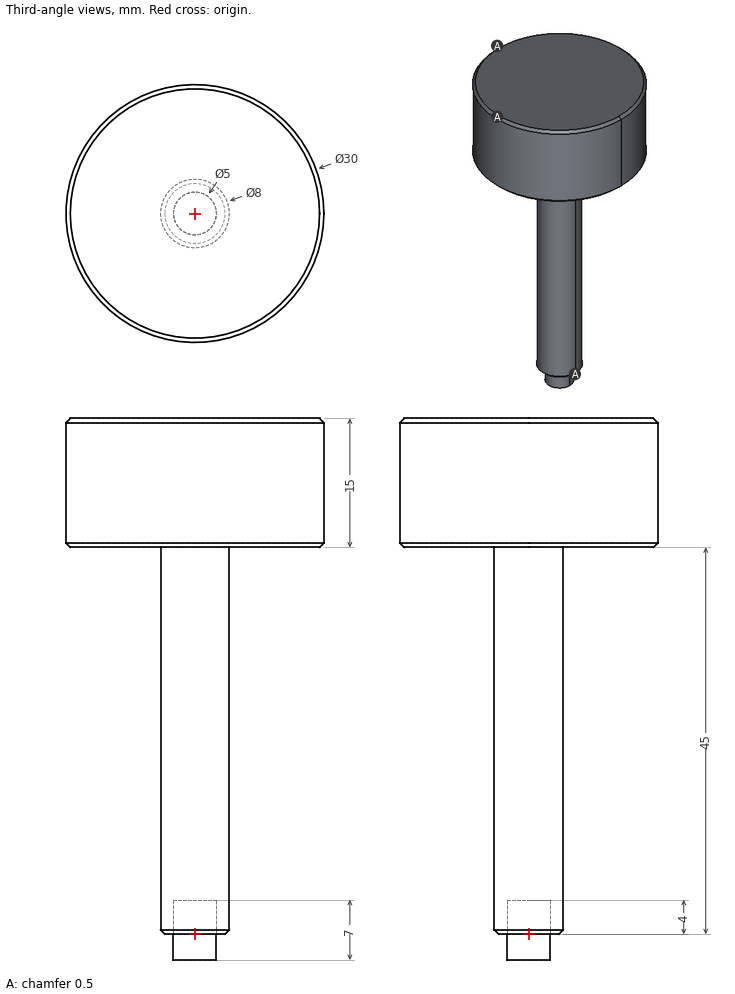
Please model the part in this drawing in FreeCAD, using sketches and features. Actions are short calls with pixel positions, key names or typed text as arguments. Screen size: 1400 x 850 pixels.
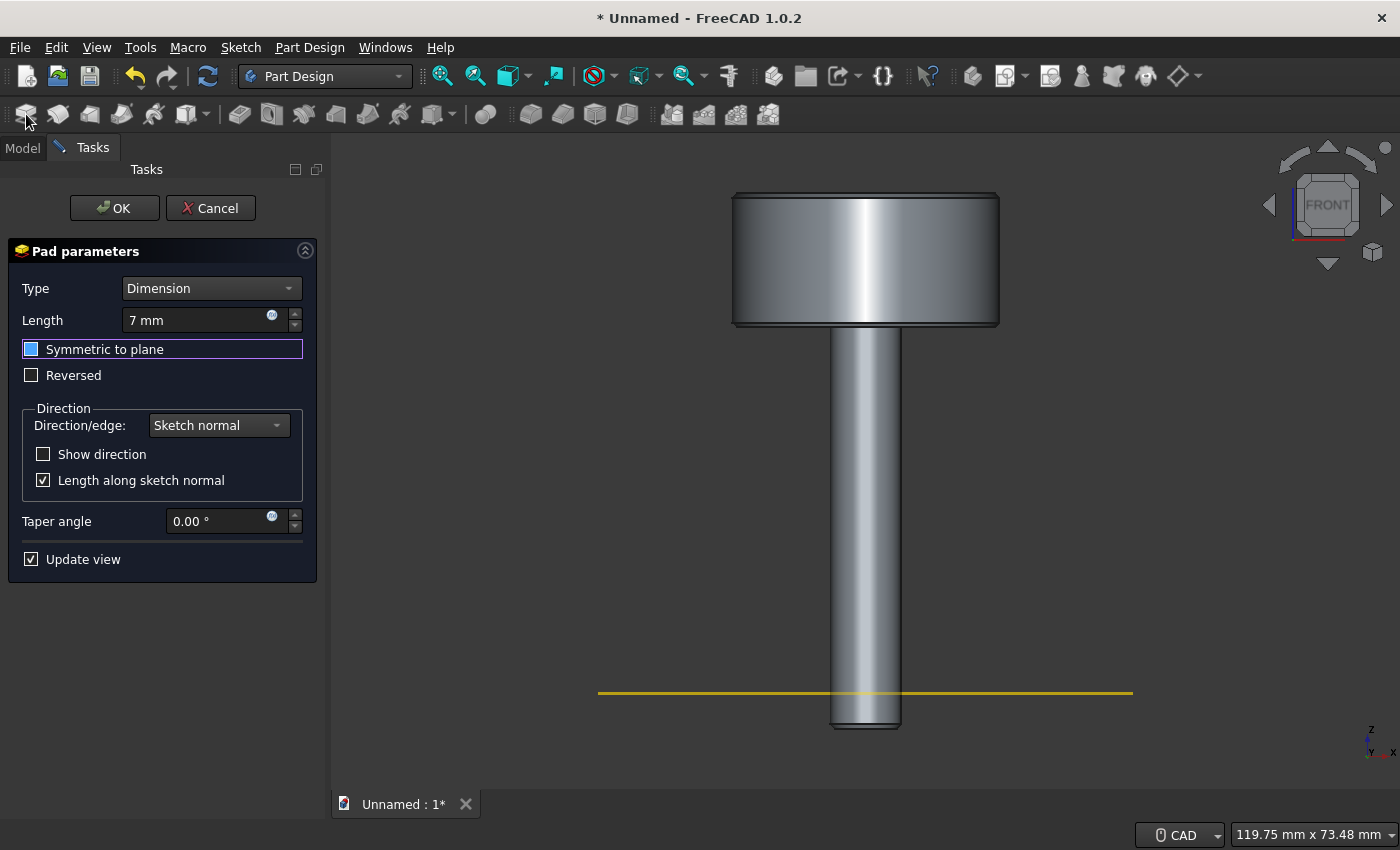
click(30, 375)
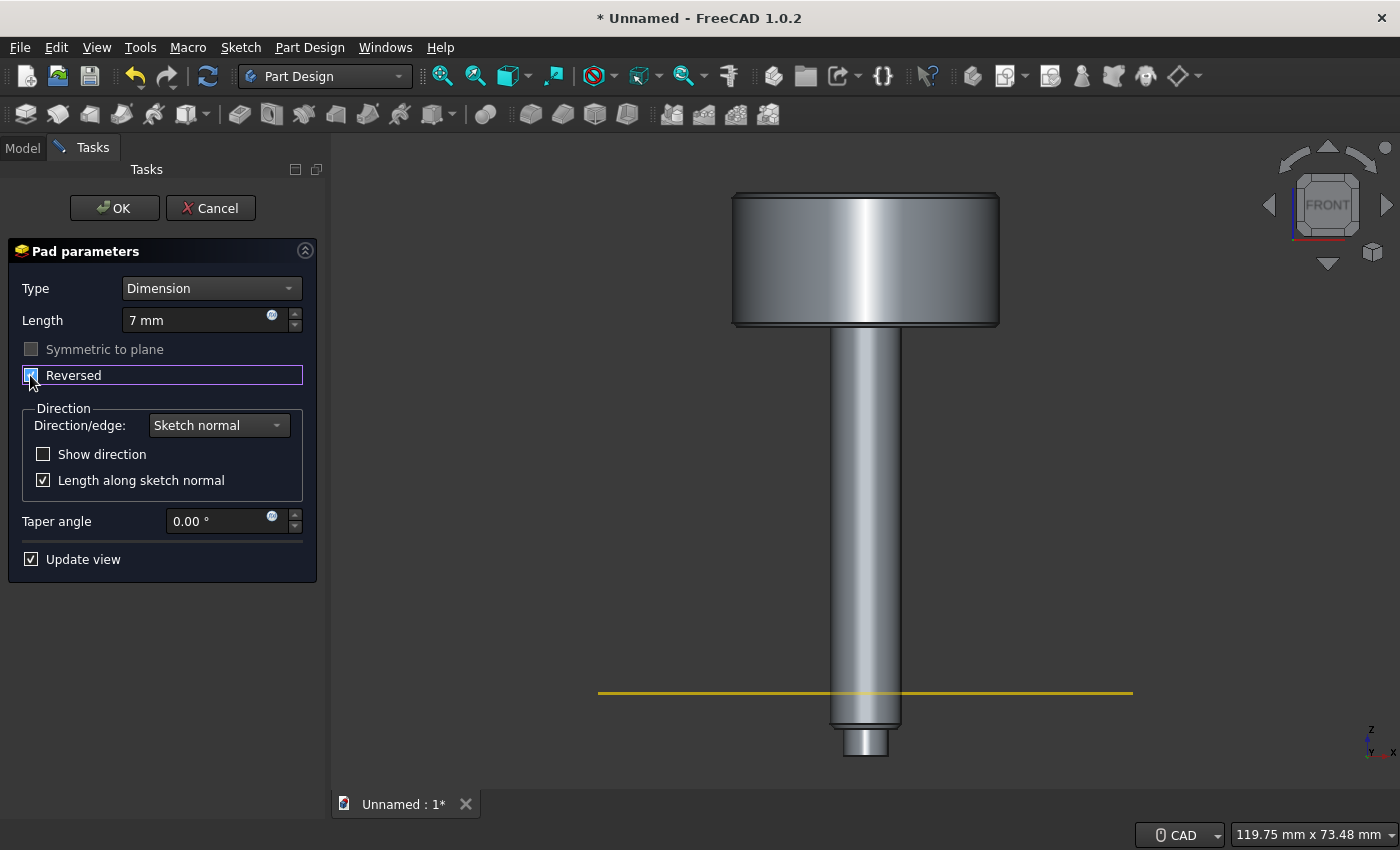
click(115, 208)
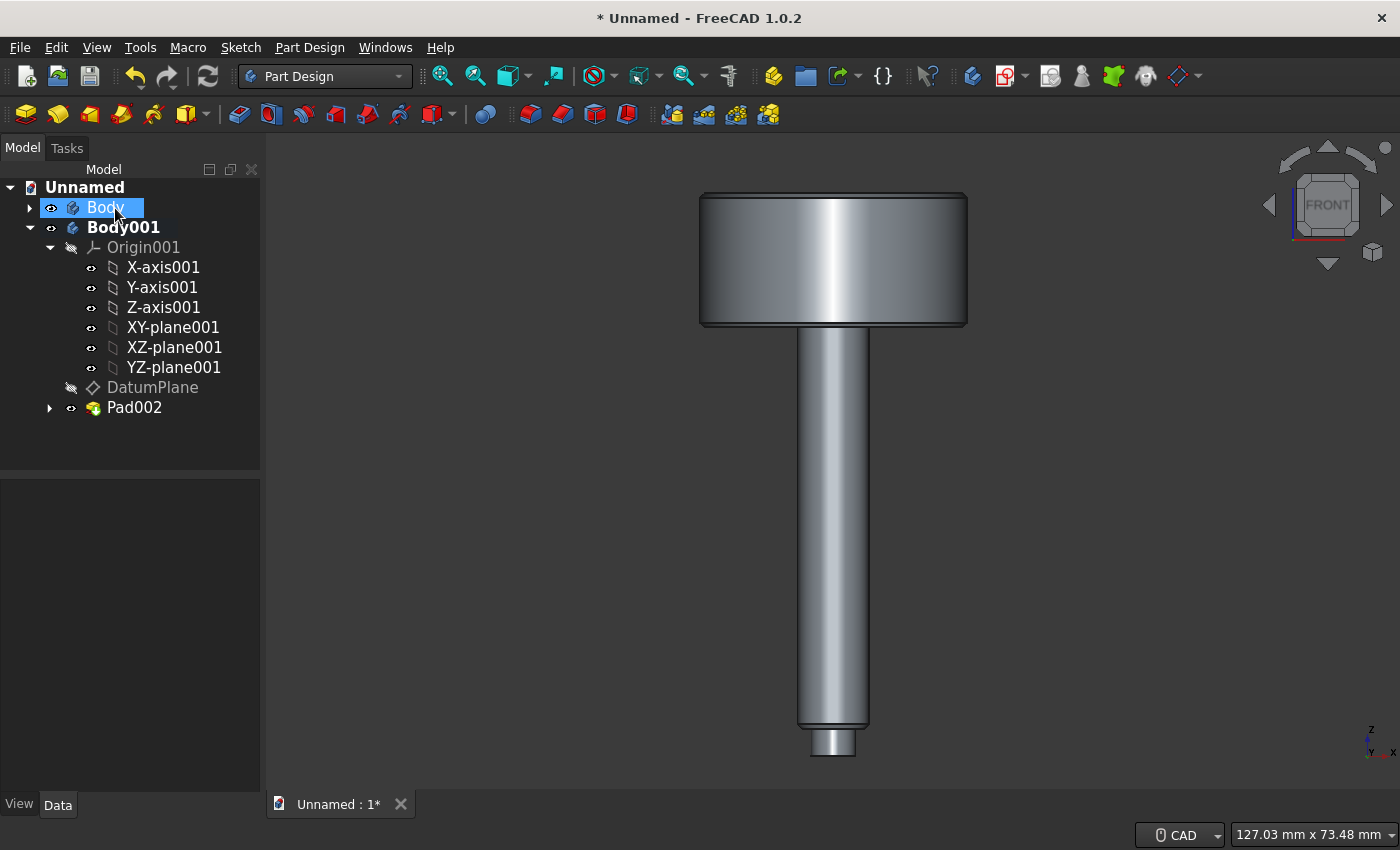
key(0)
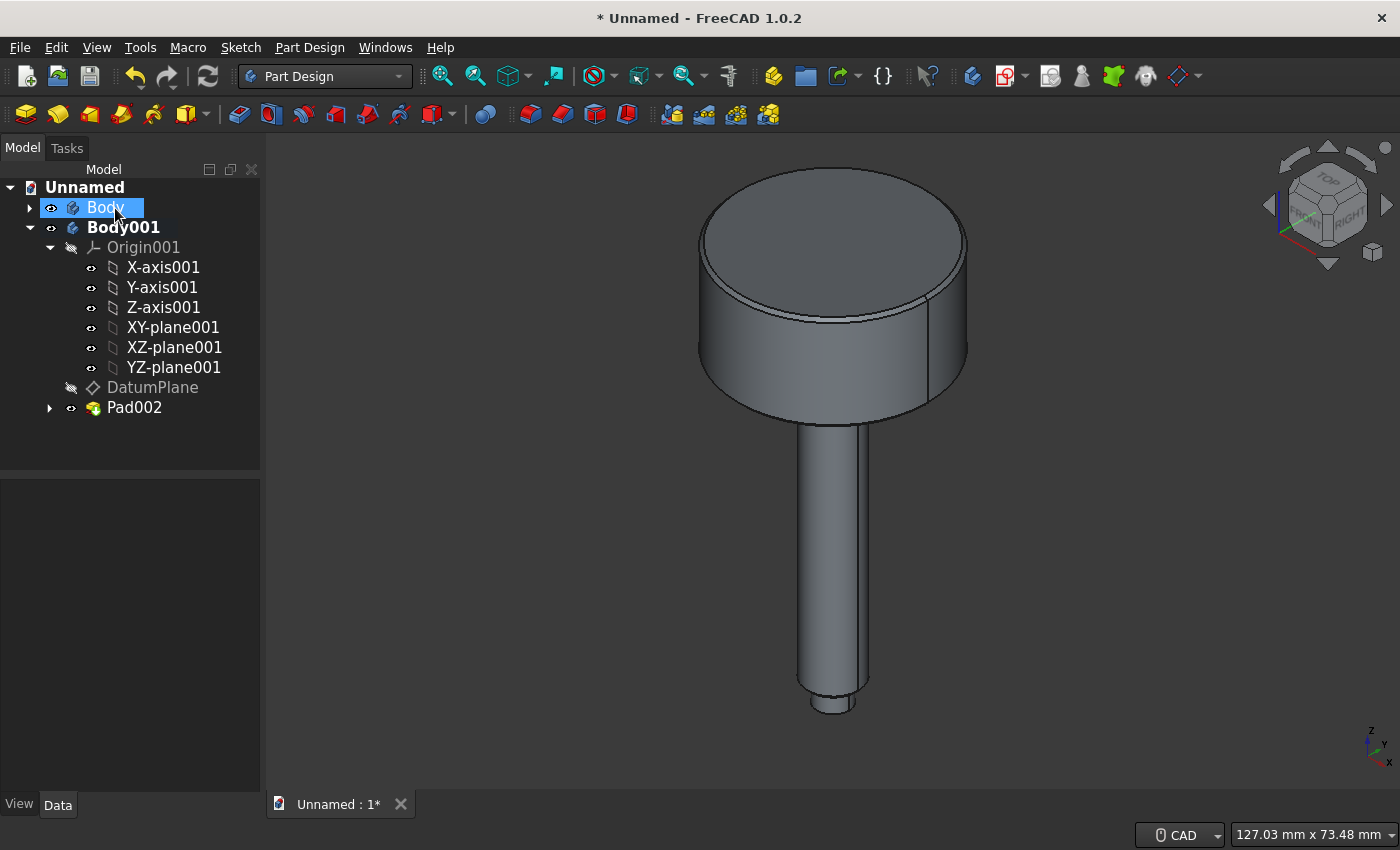
click(444, 76)